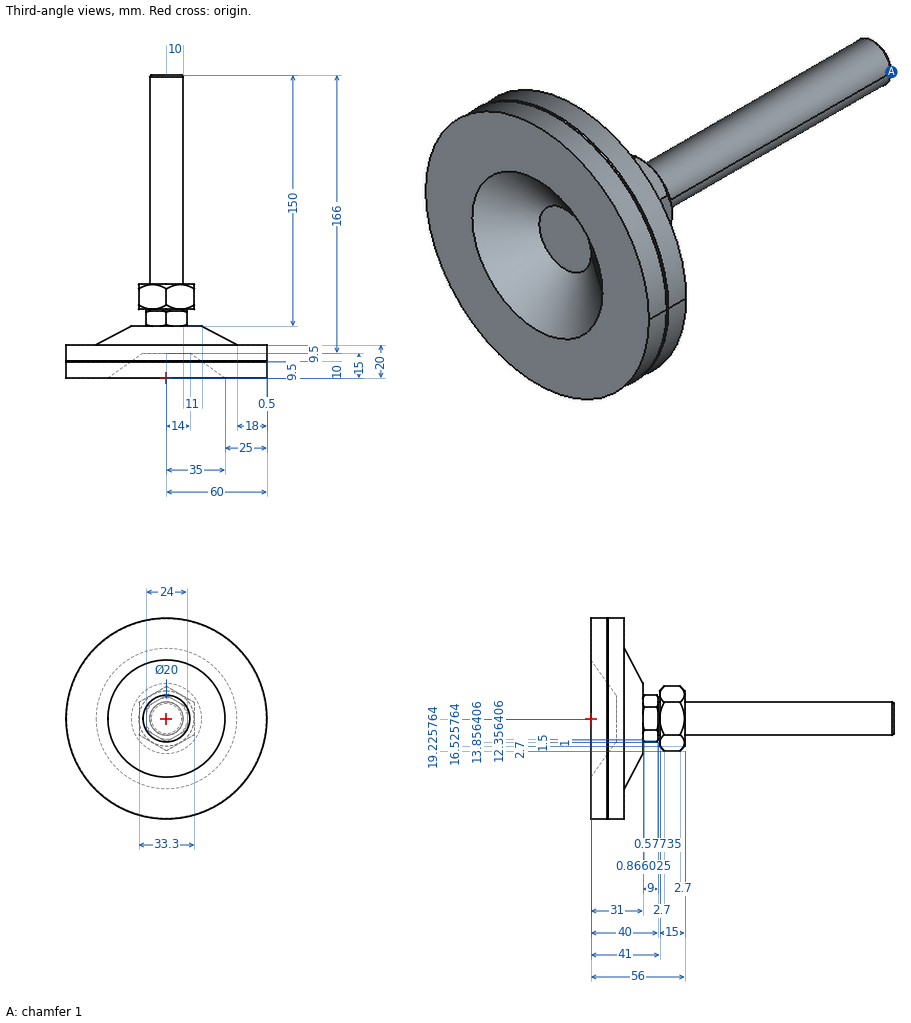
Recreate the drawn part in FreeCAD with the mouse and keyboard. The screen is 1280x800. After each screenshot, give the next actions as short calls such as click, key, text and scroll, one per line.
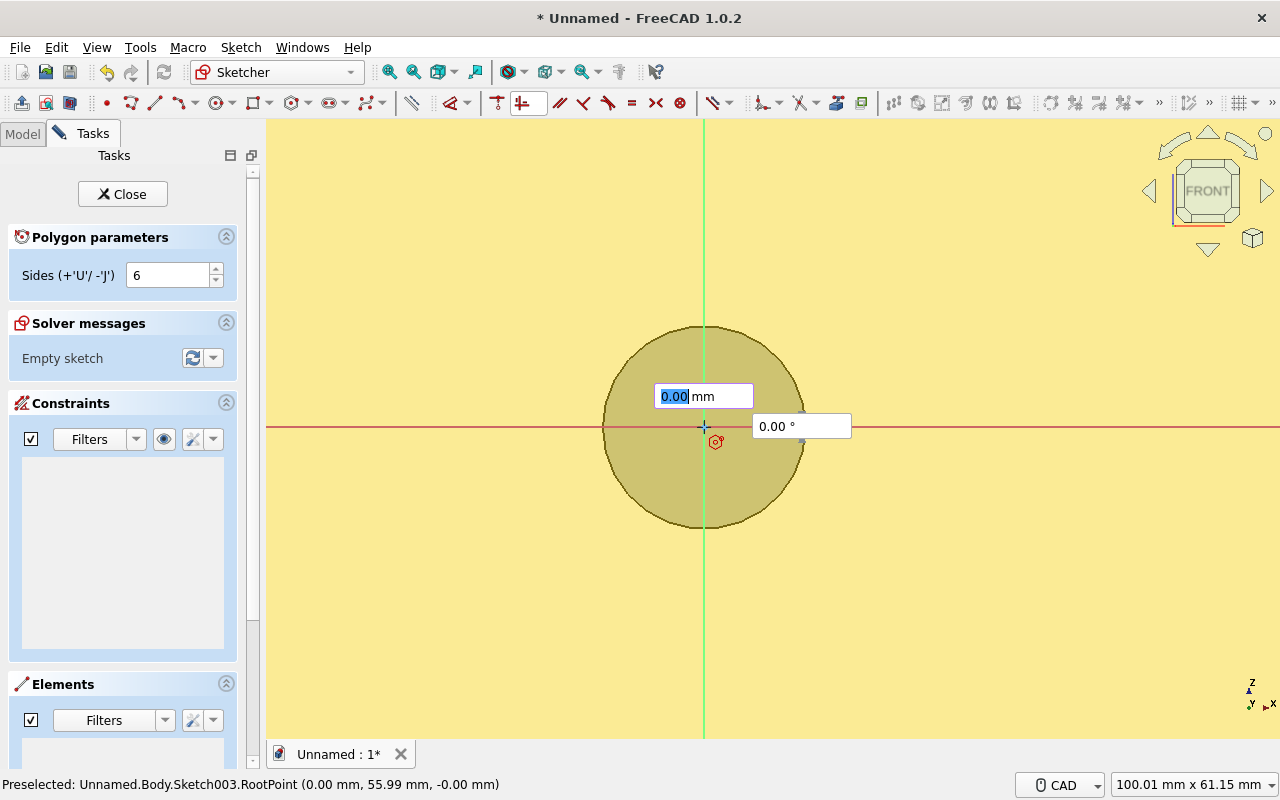
click(704, 233)
right_click(704, 233)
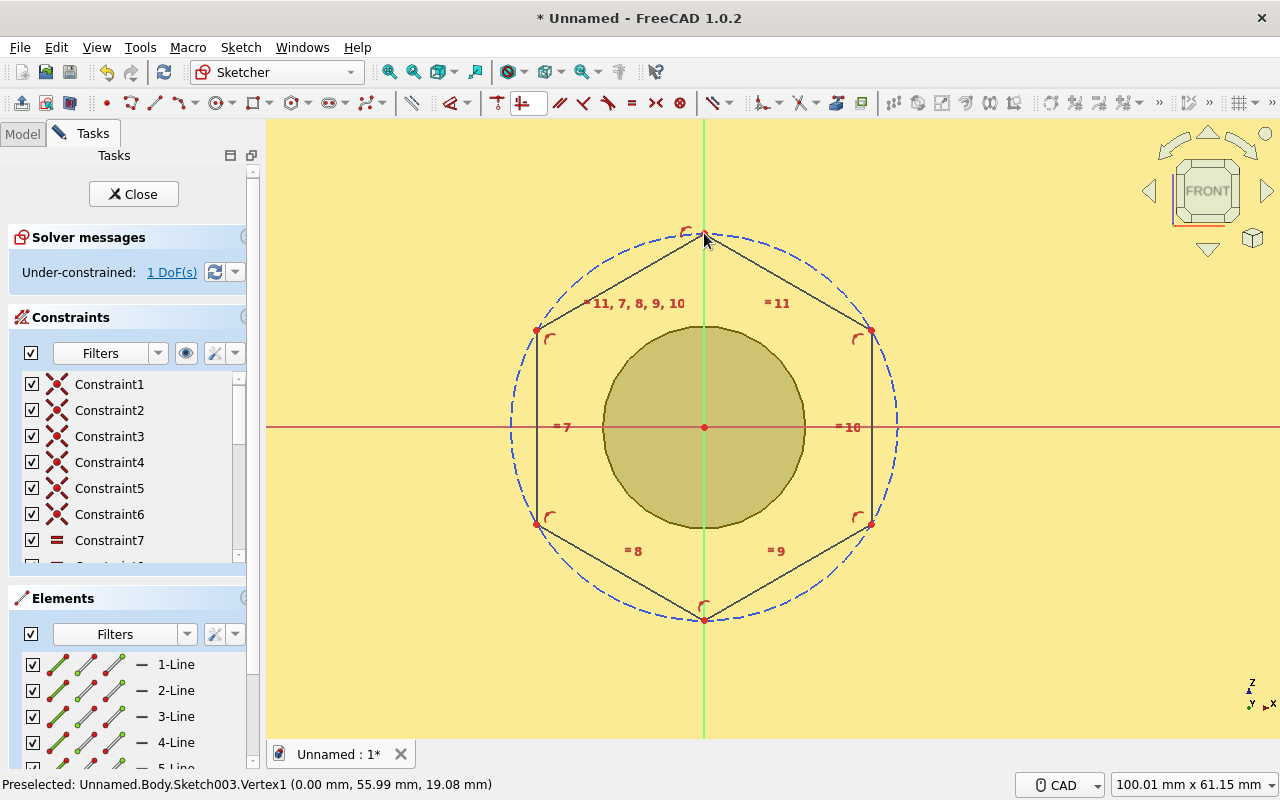
click(216, 104)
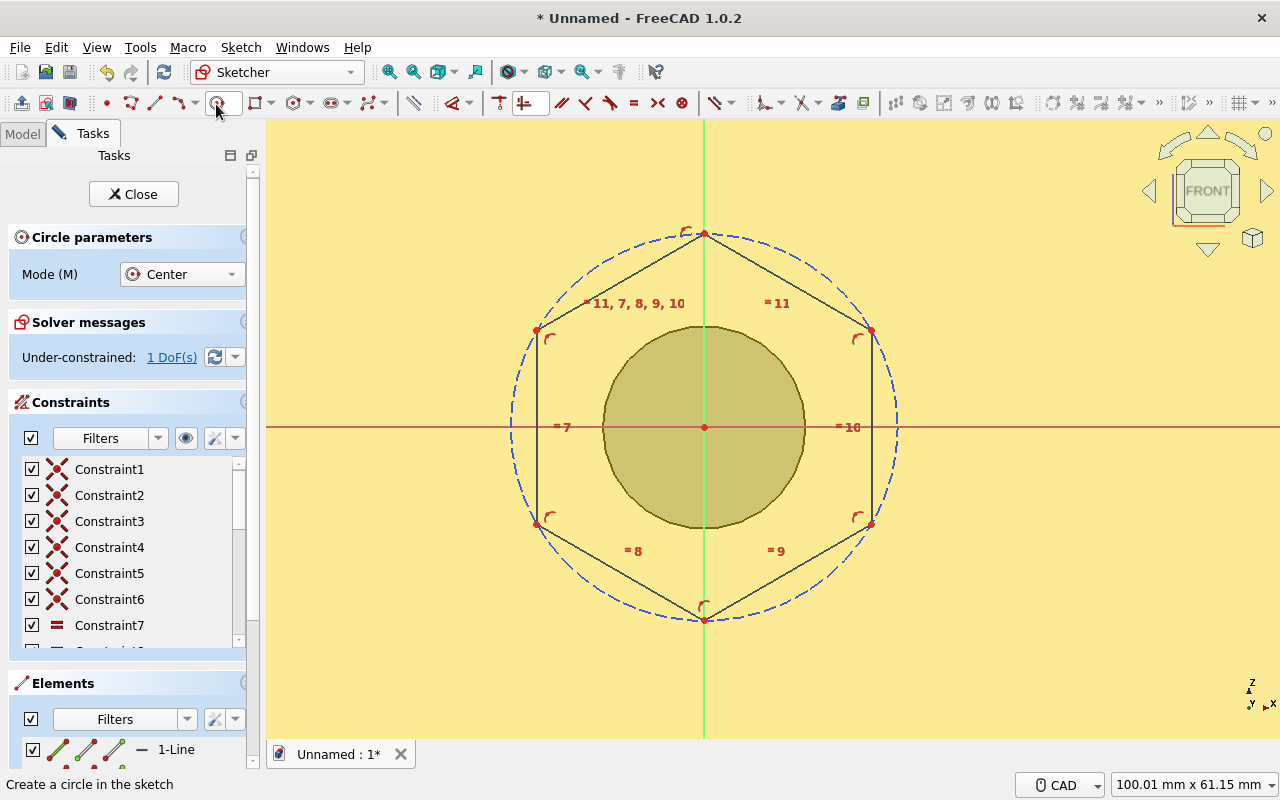
click(704, 427)
move(776, 356)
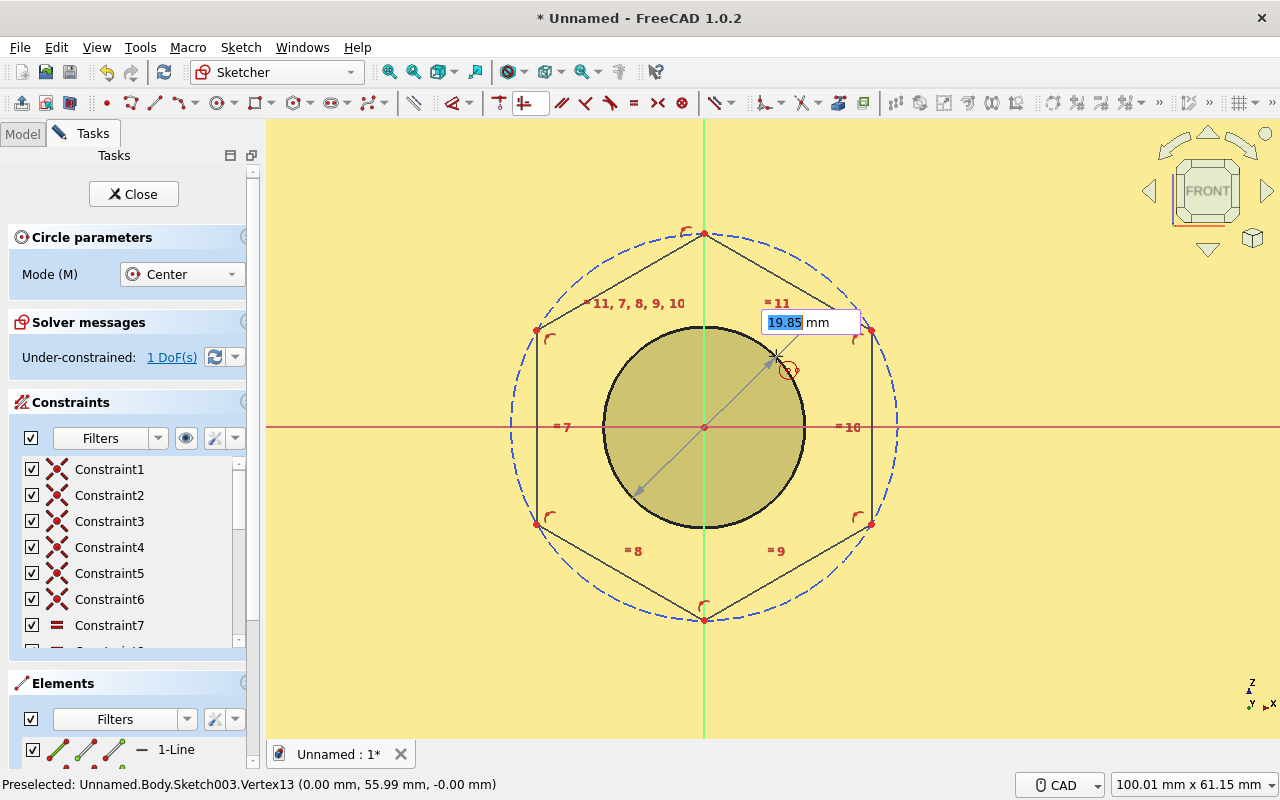
text(20)
key(Return)
key(Escape)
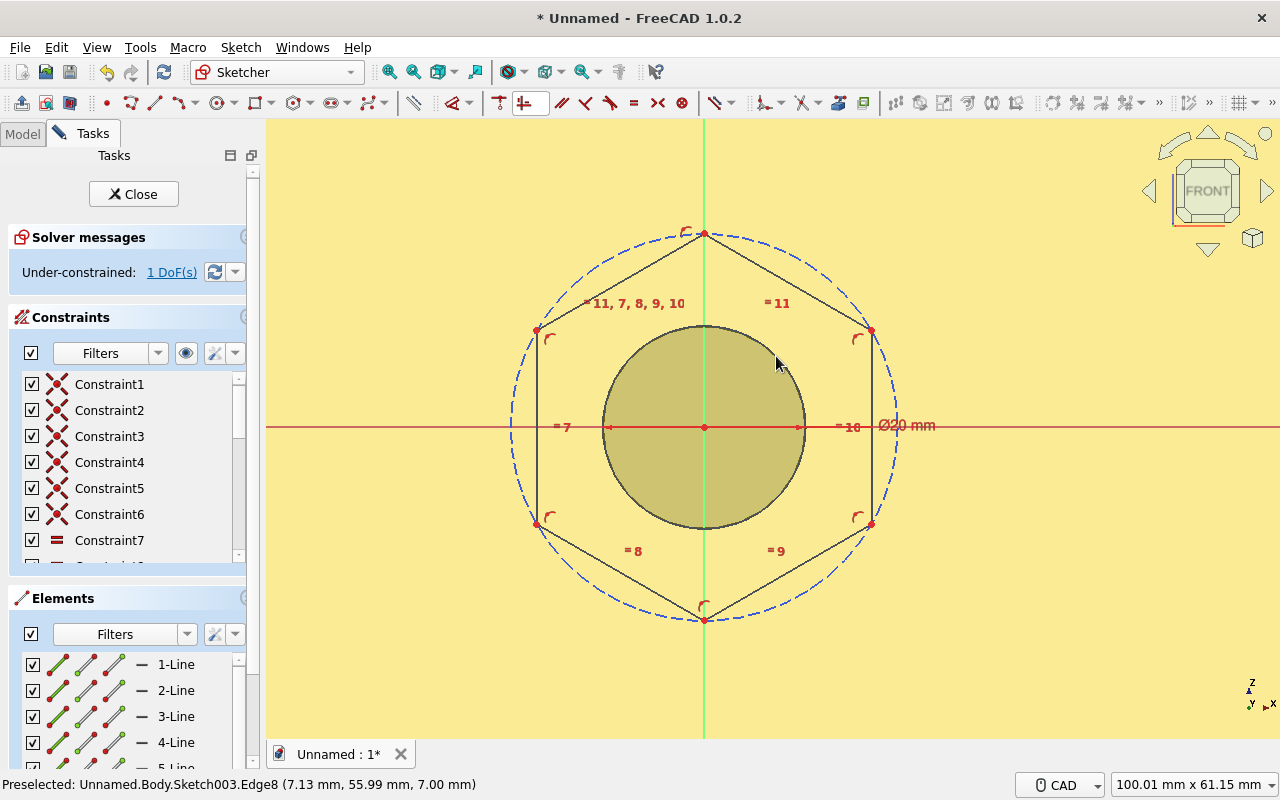
click(452, 104)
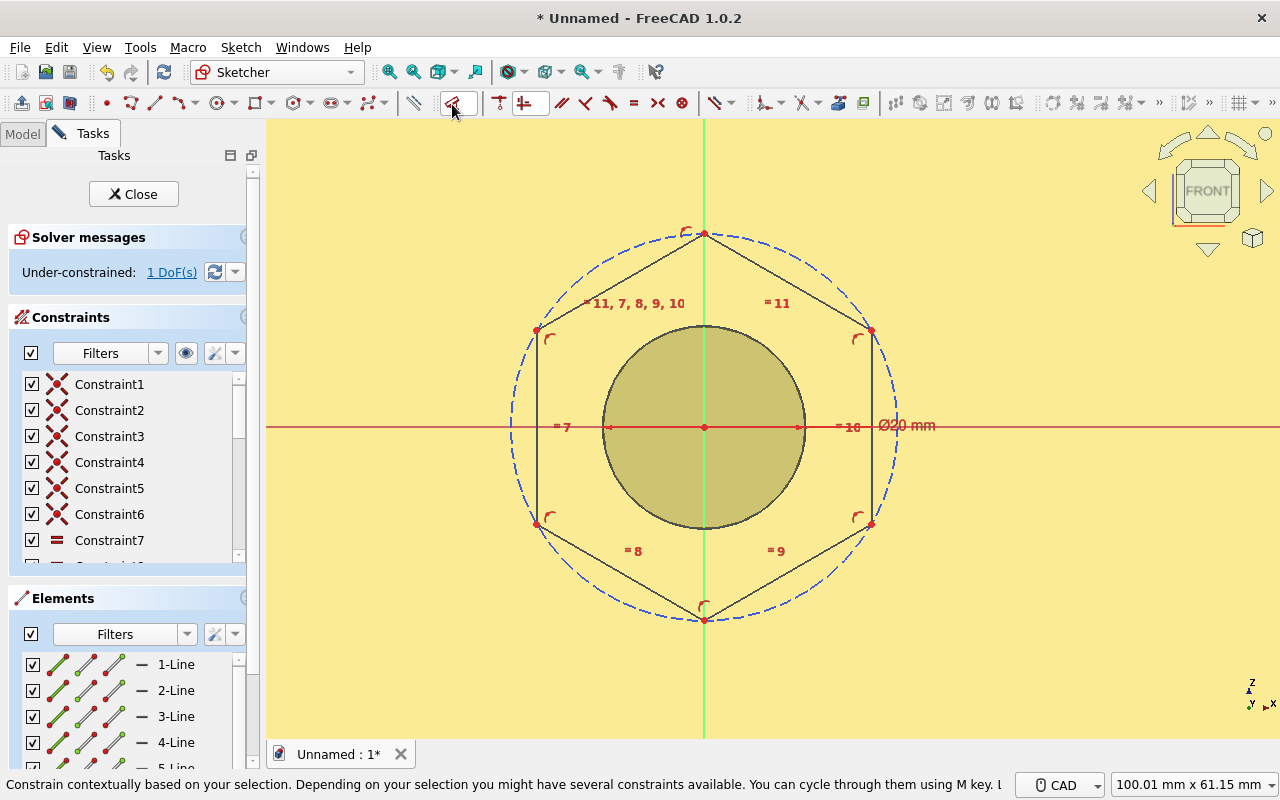
click(537, 331)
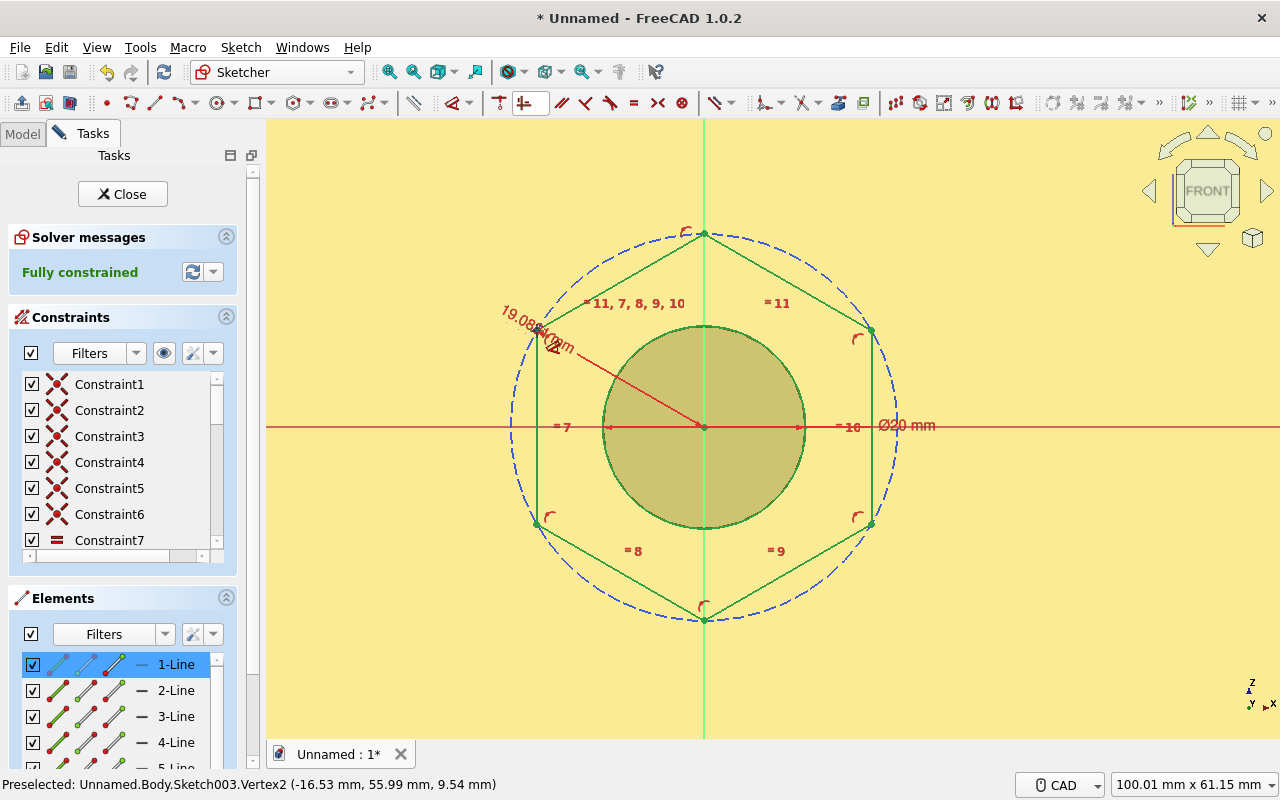
click(872, 524)
click(627, 558)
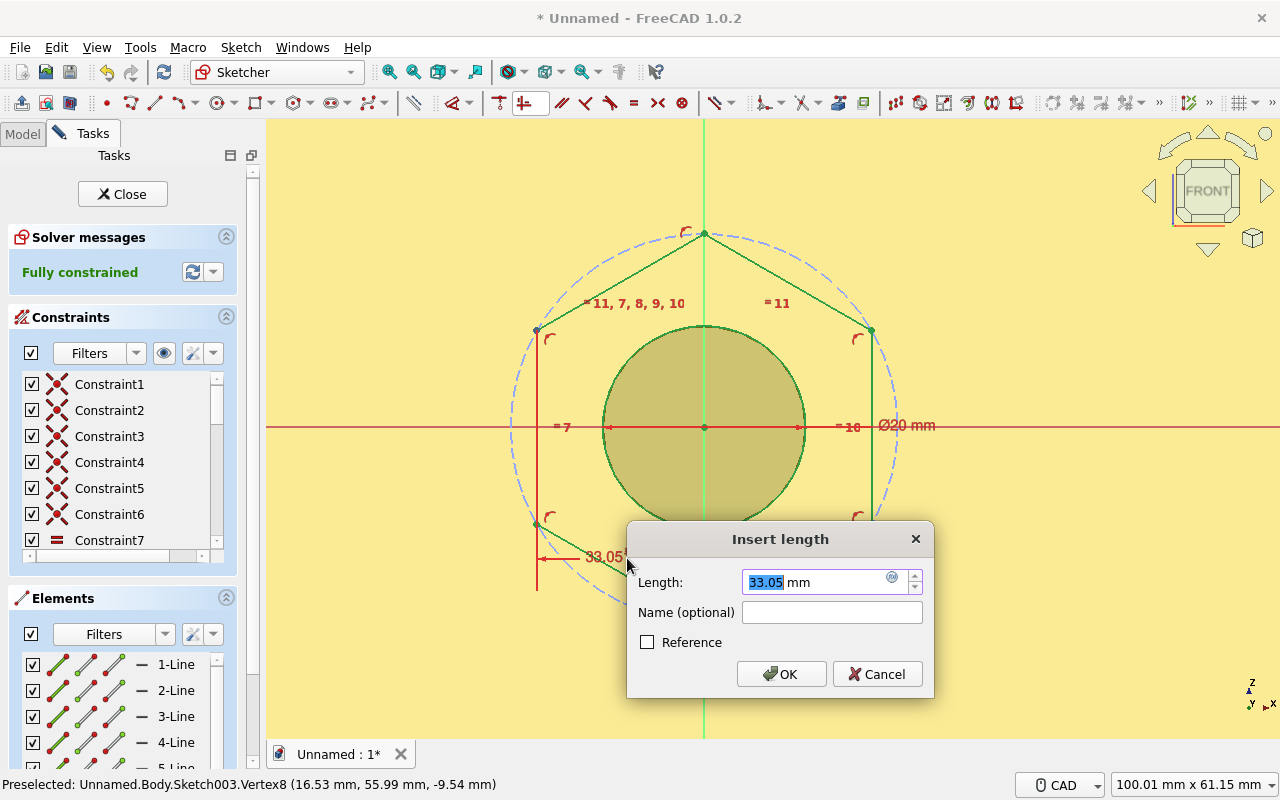
text(33.3)
key(Return)
key(Escape)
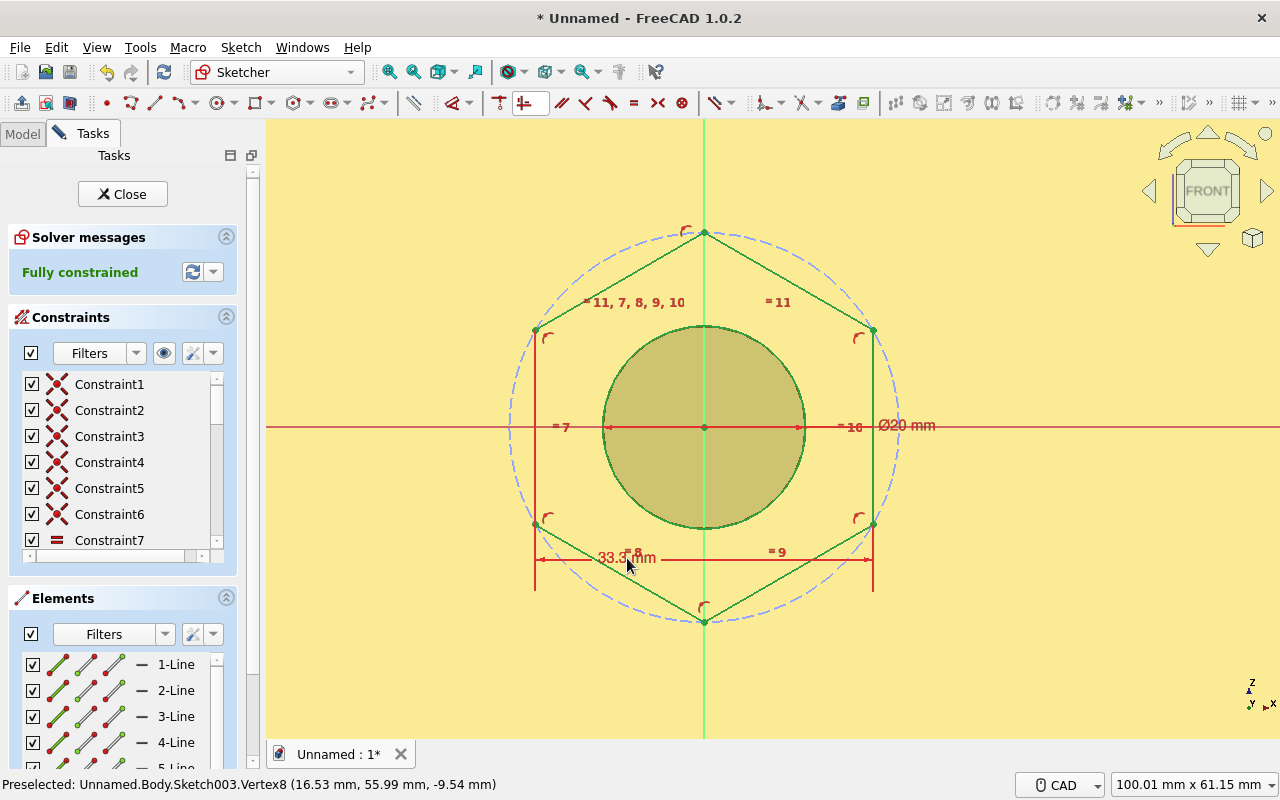
click(123, 194)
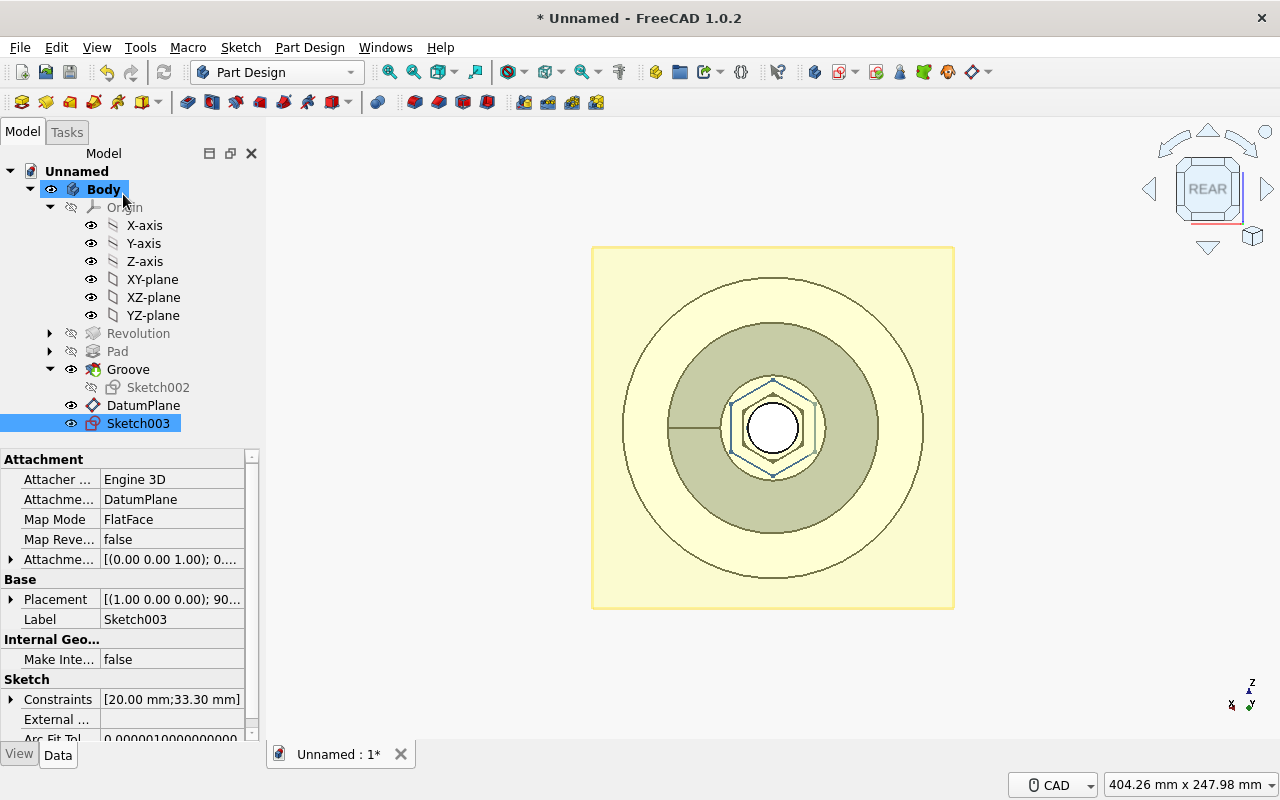
click(22, 102)